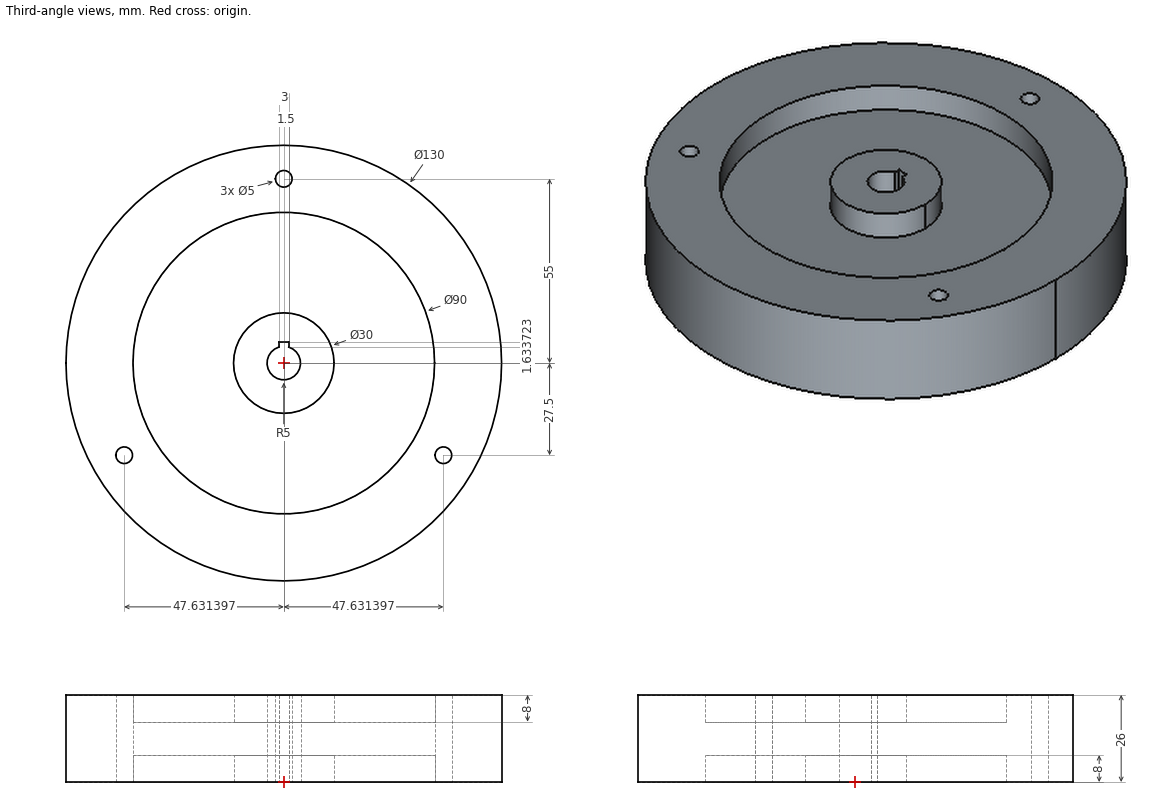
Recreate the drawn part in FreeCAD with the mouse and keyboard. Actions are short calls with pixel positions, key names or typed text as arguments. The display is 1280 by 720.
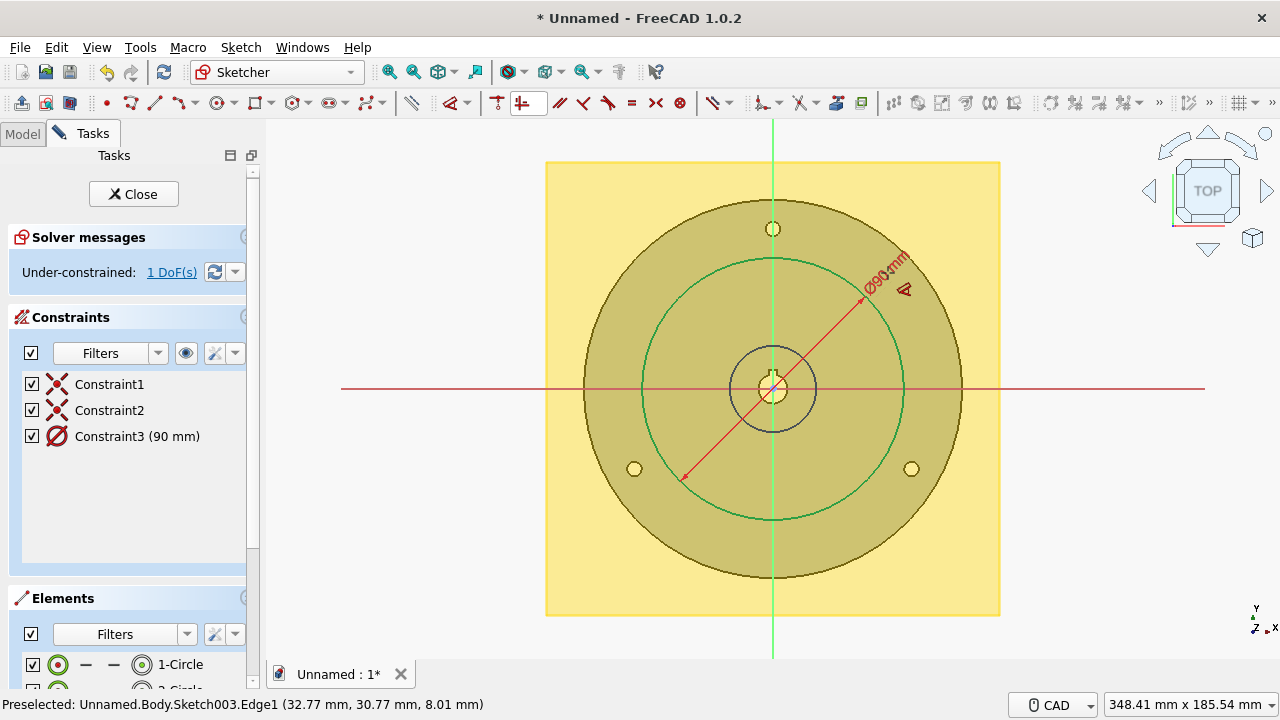
click(803, 358)
click(825, 335)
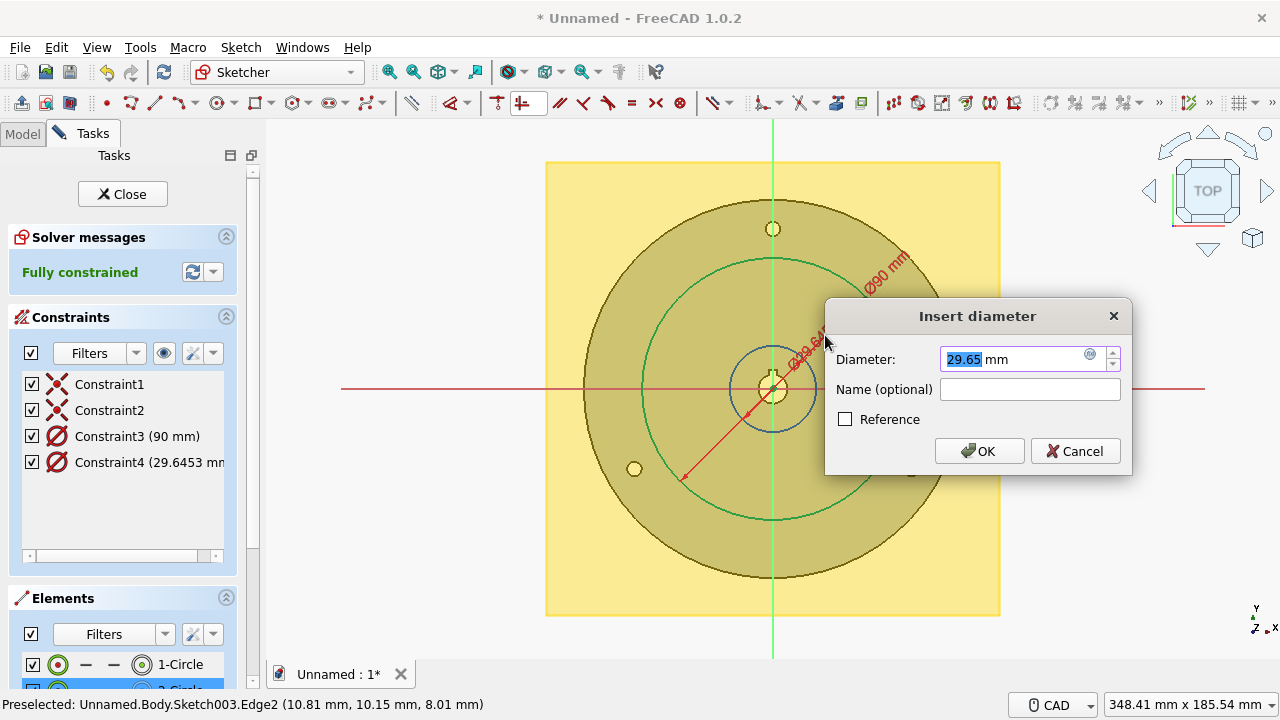
text(30)
key(Return)
key(Escape)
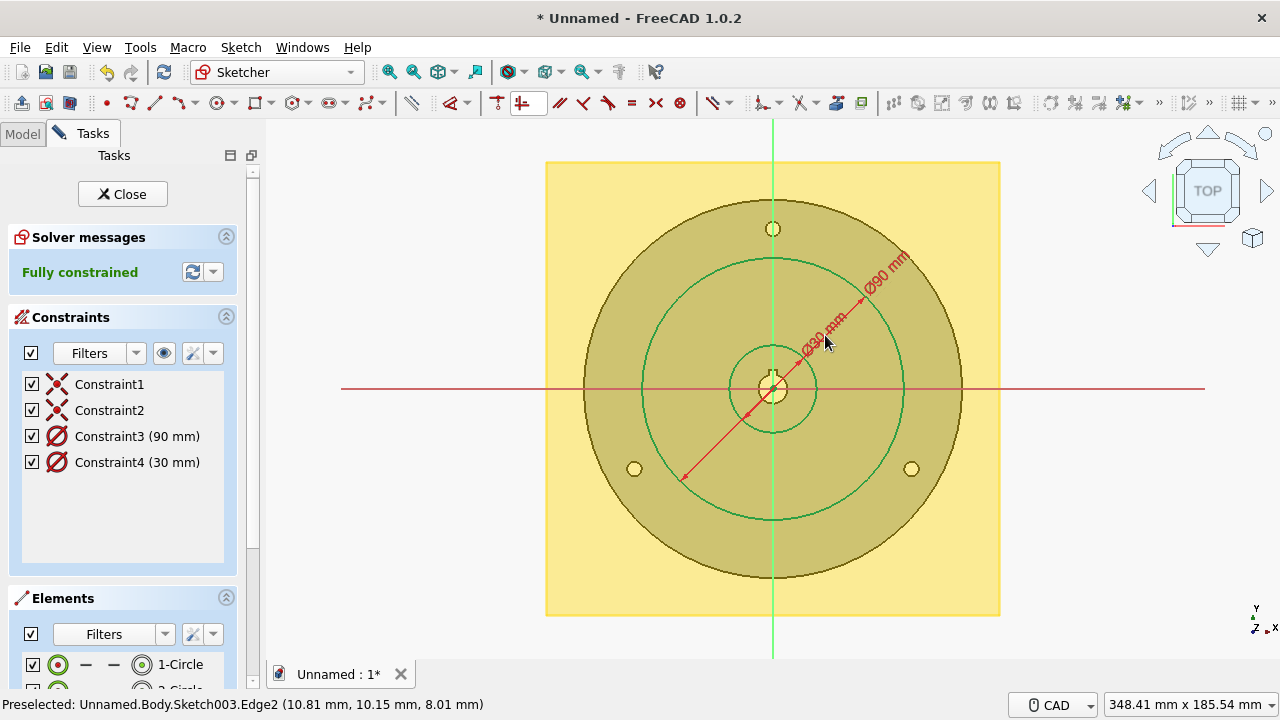
click(123, 194)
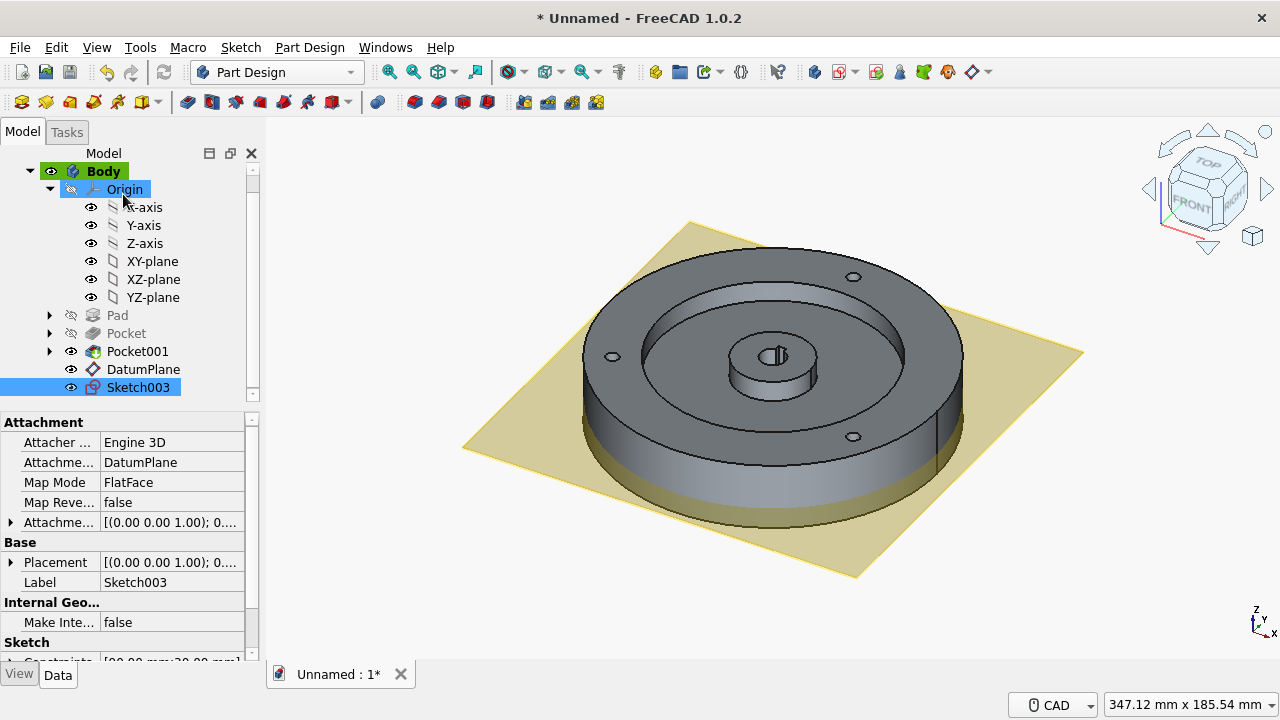
click(188, 102)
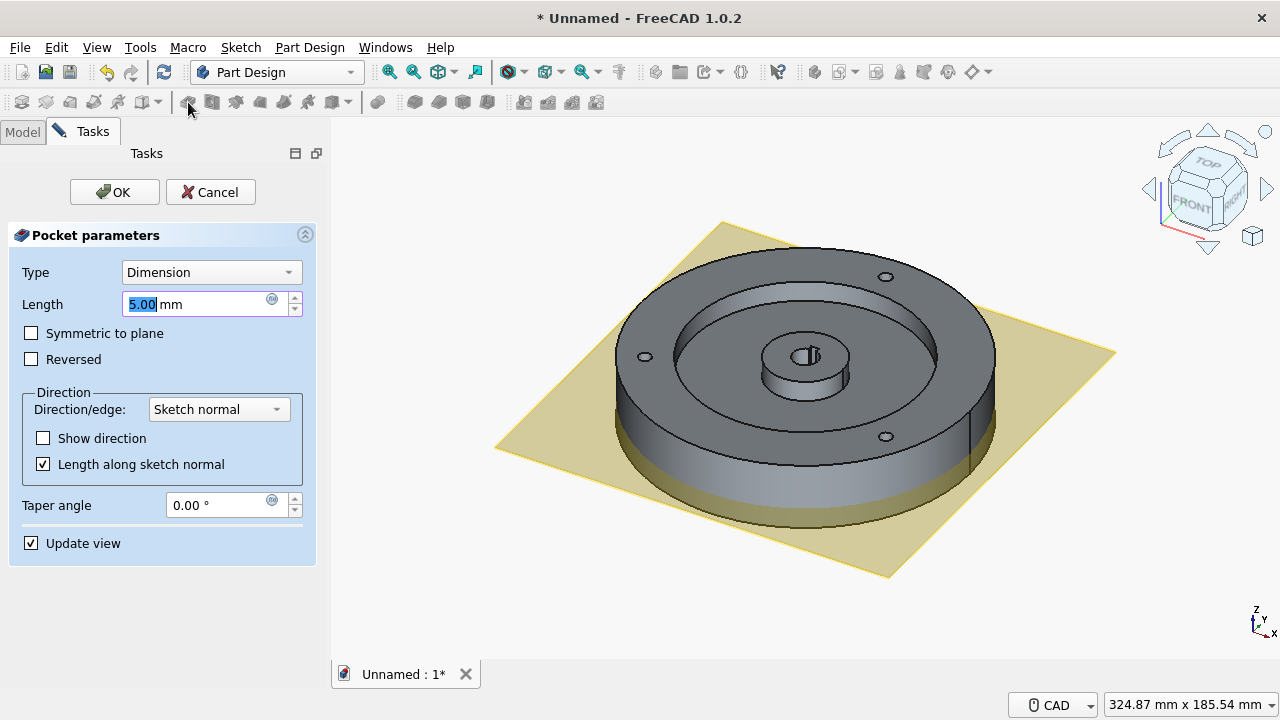
text(8)
key(Tab)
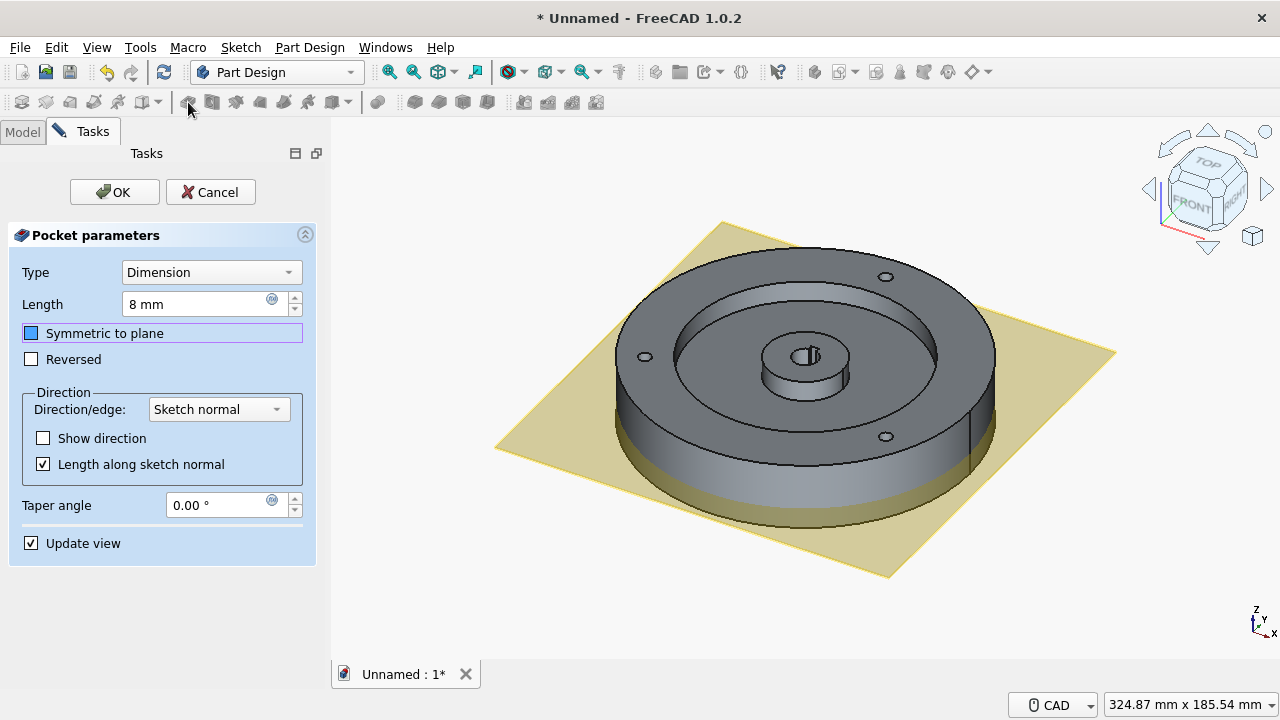
click(115, 192)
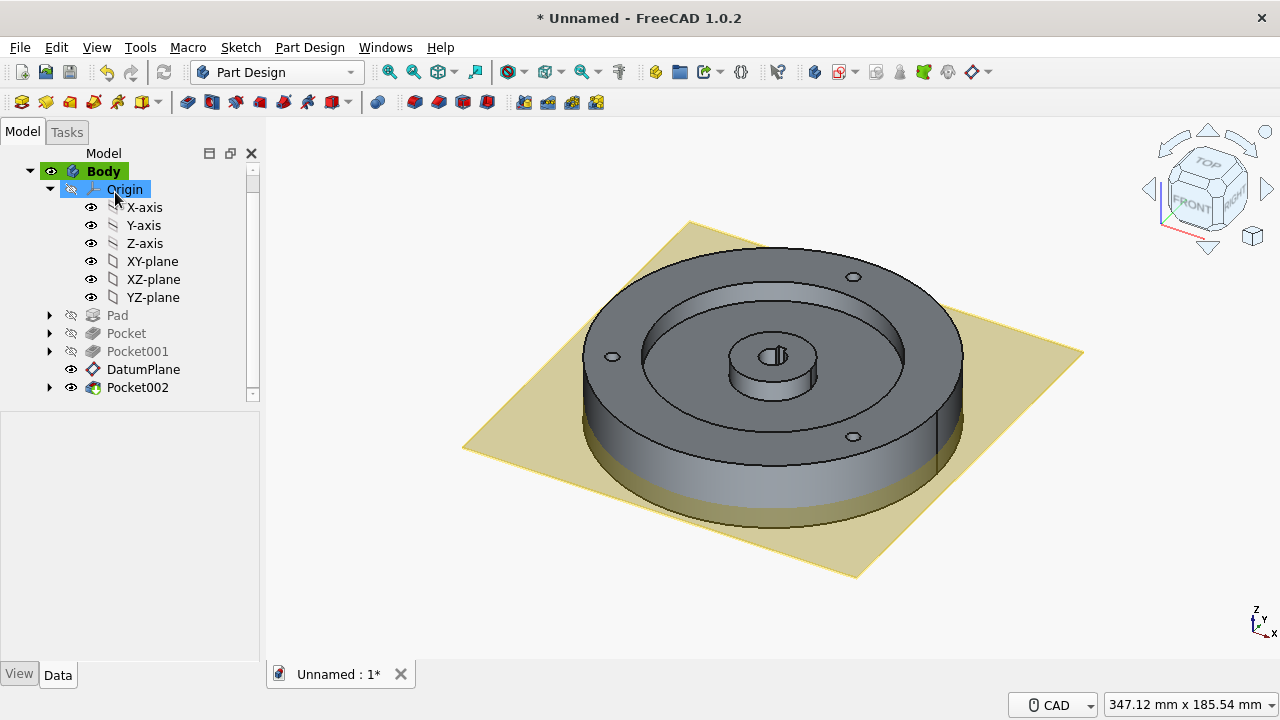
click(116, 369)
key(space)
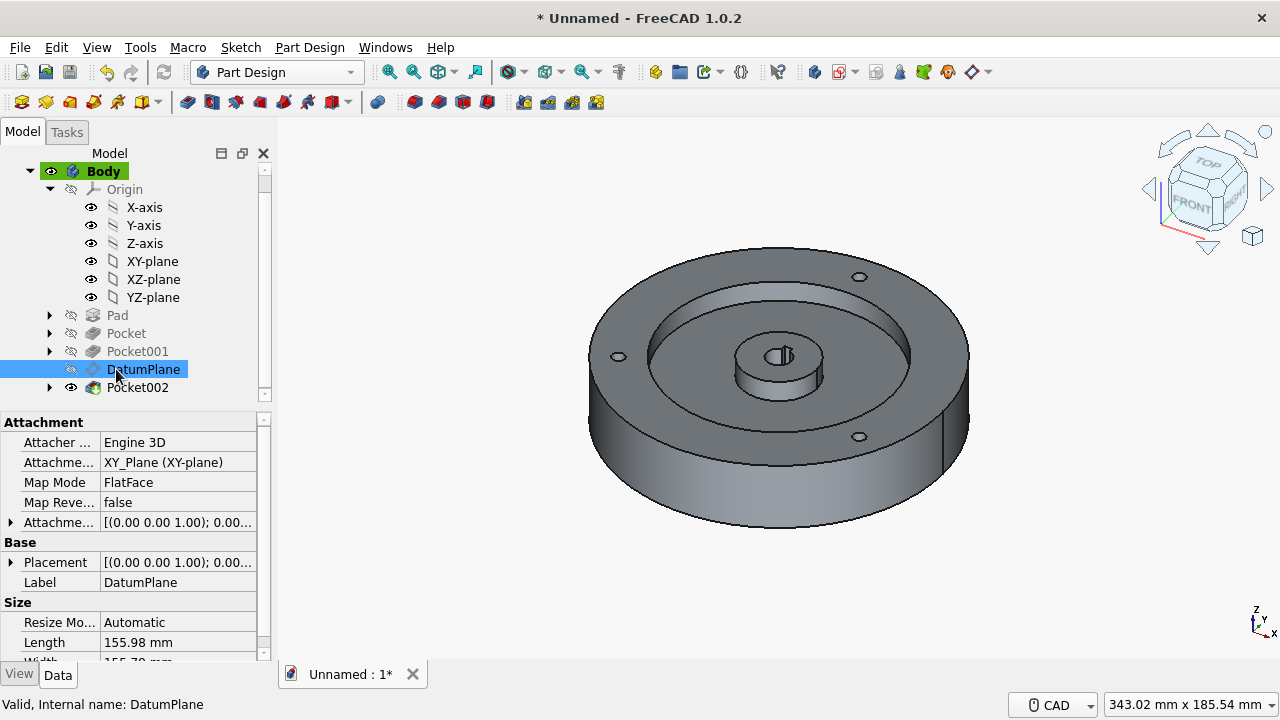
key(0)